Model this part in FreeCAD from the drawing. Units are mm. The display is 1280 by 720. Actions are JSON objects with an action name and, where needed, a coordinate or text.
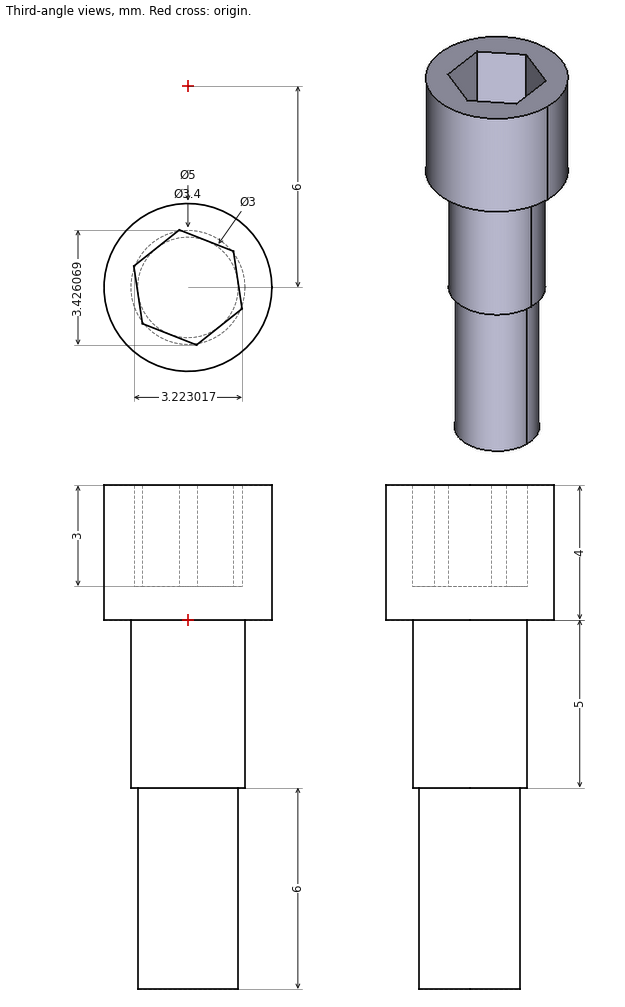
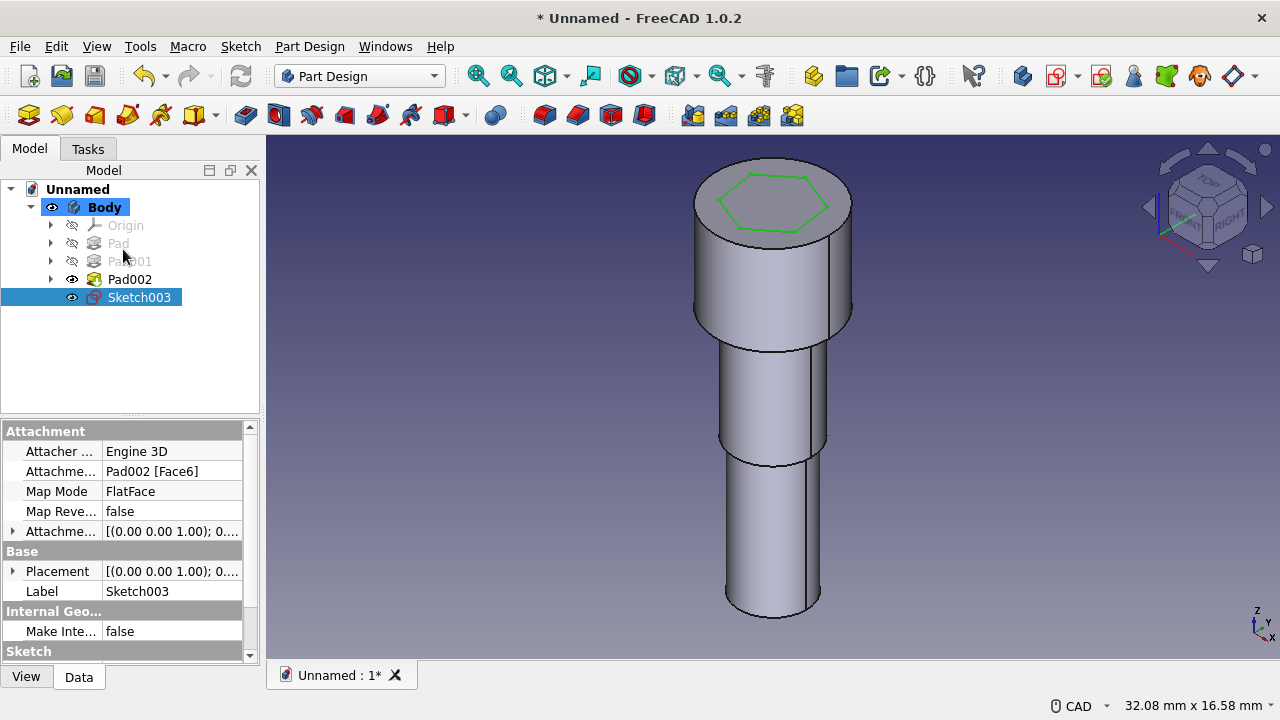
{"action": "left_click", "coordinate": [246, 116]}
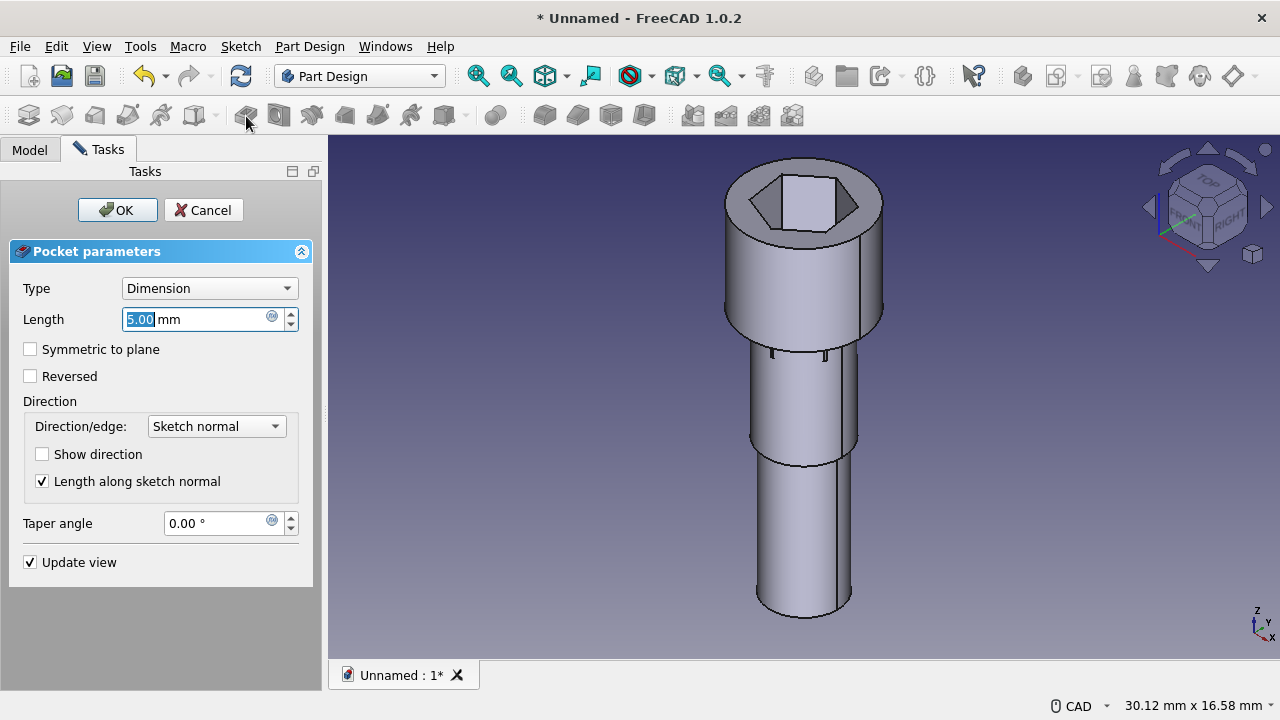
{"action": "type", "text": "3"}
{"action": "key", "text": "Tab"}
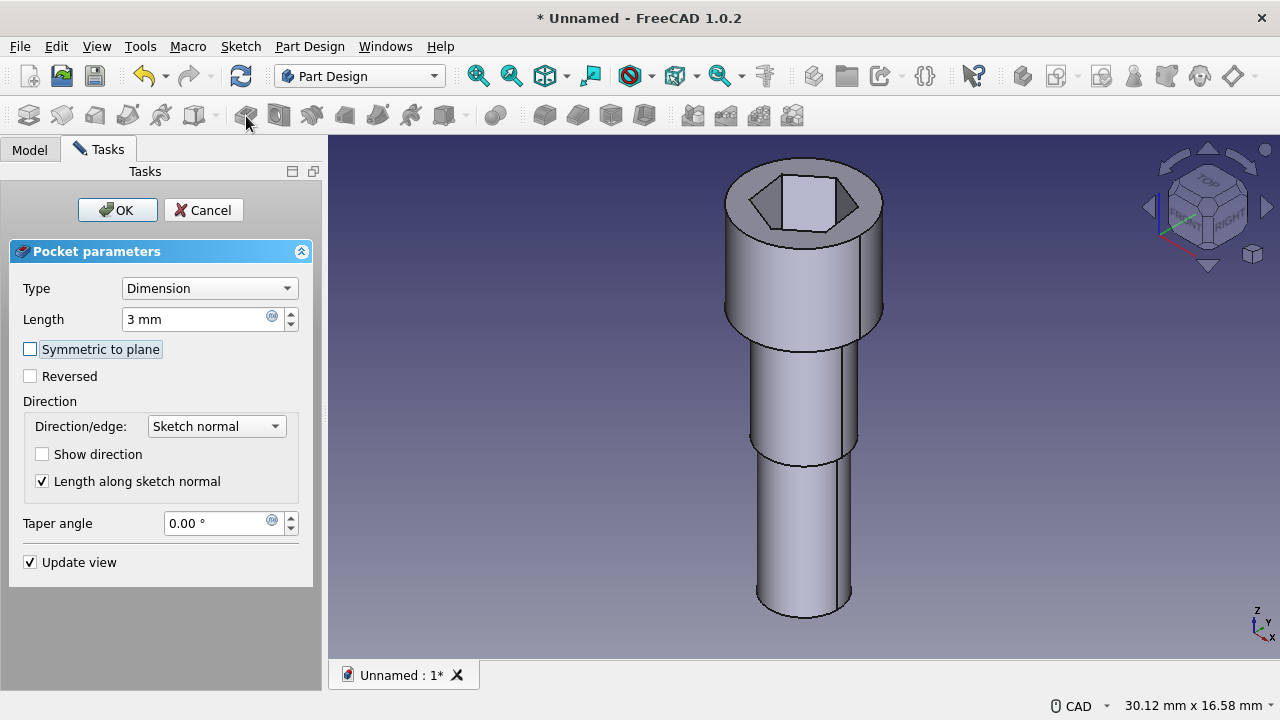
{"action": "left_click", "coordinate": [118, 210]}